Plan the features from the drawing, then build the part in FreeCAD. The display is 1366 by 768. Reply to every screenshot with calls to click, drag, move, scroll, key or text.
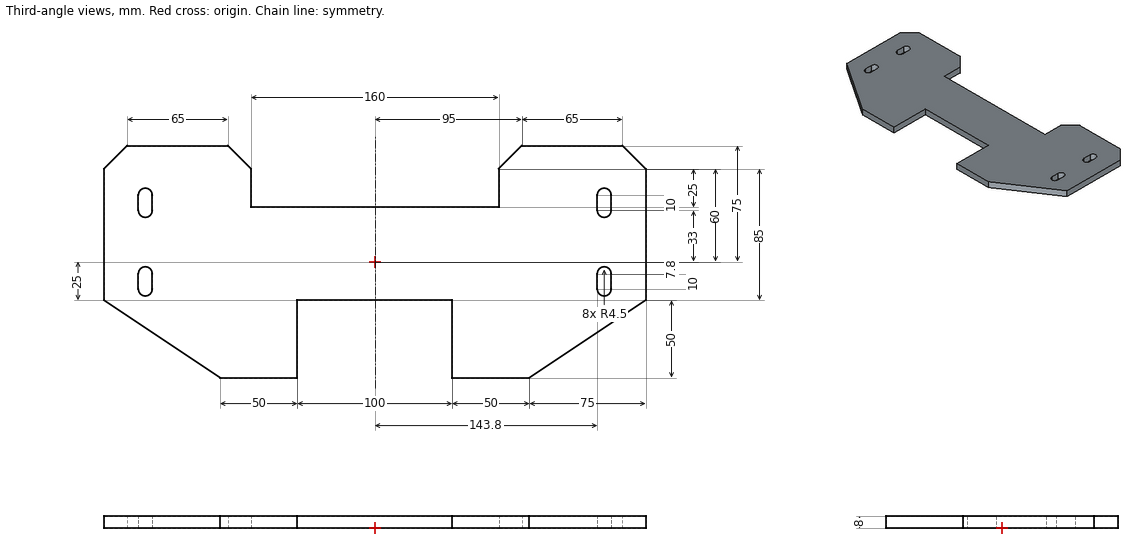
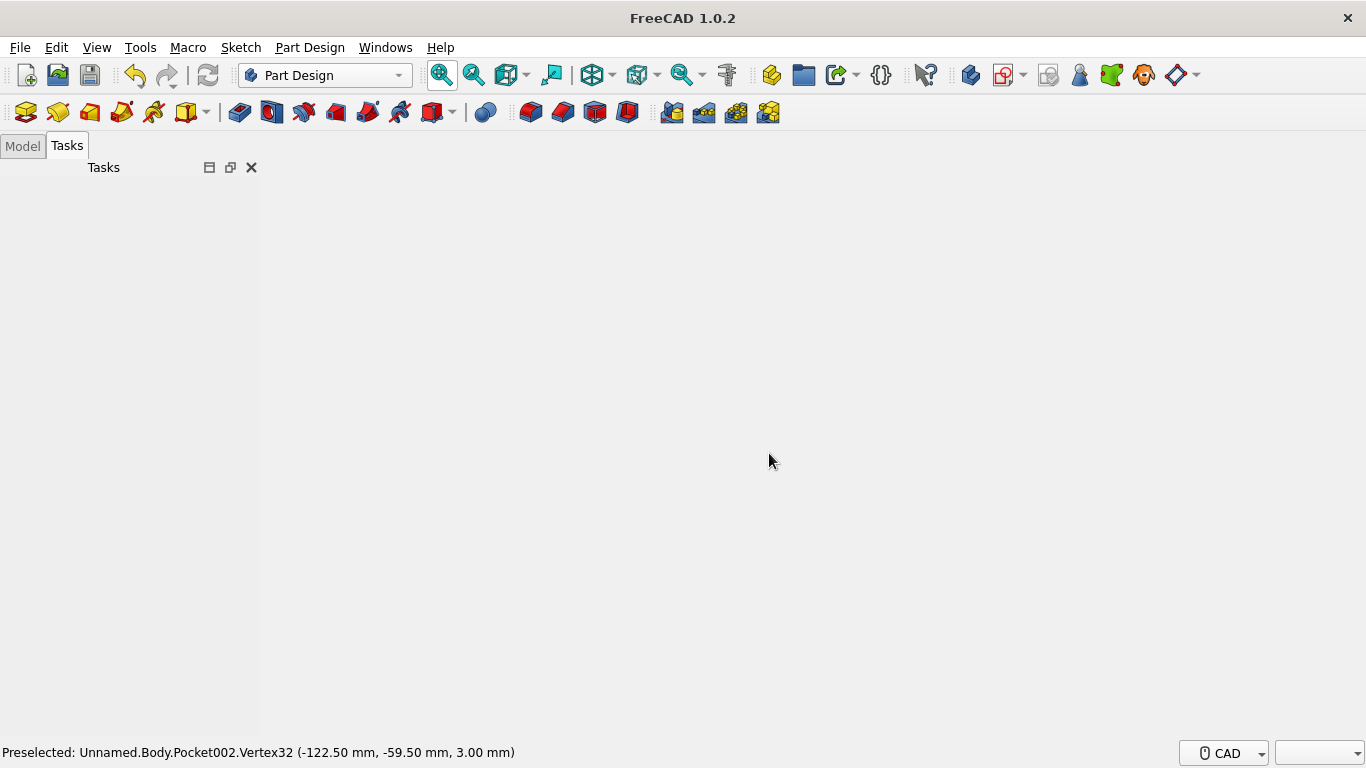
click(26, 76)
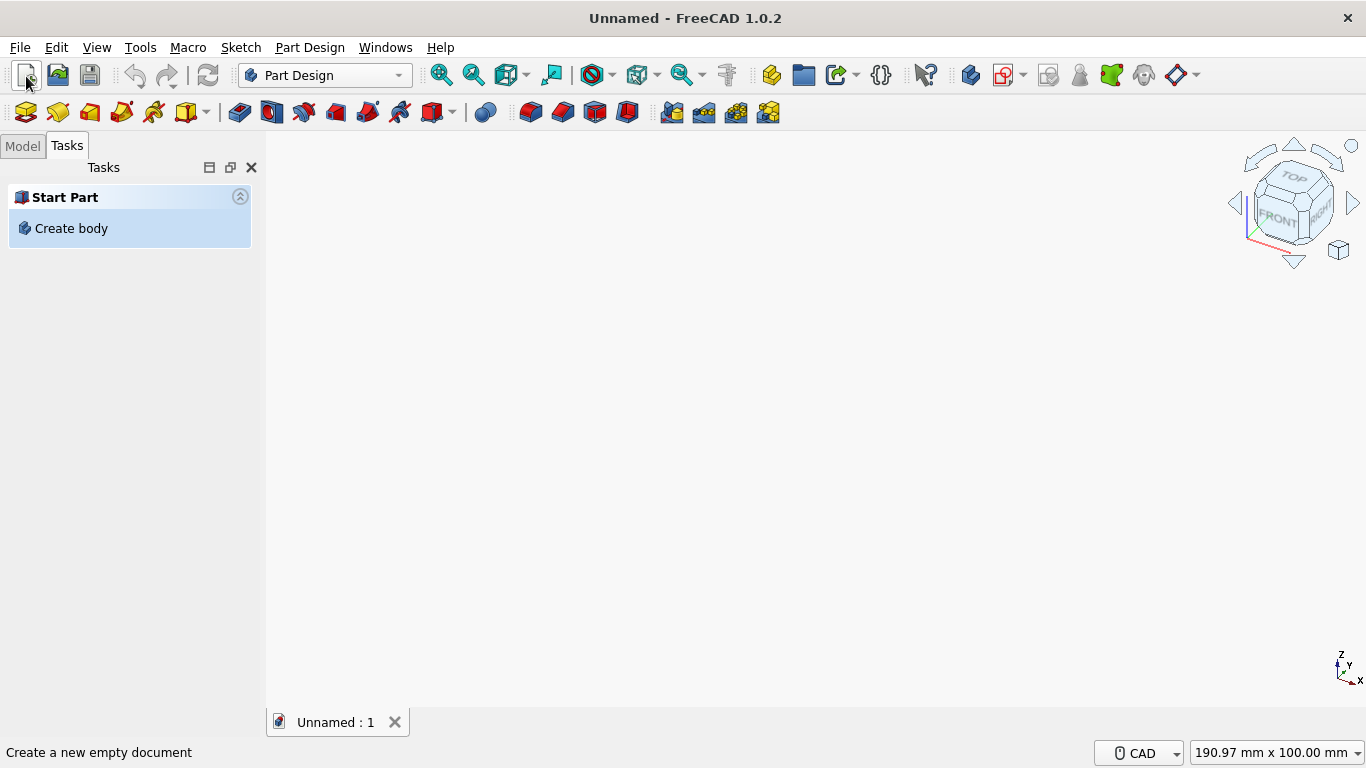
click(1004, 76)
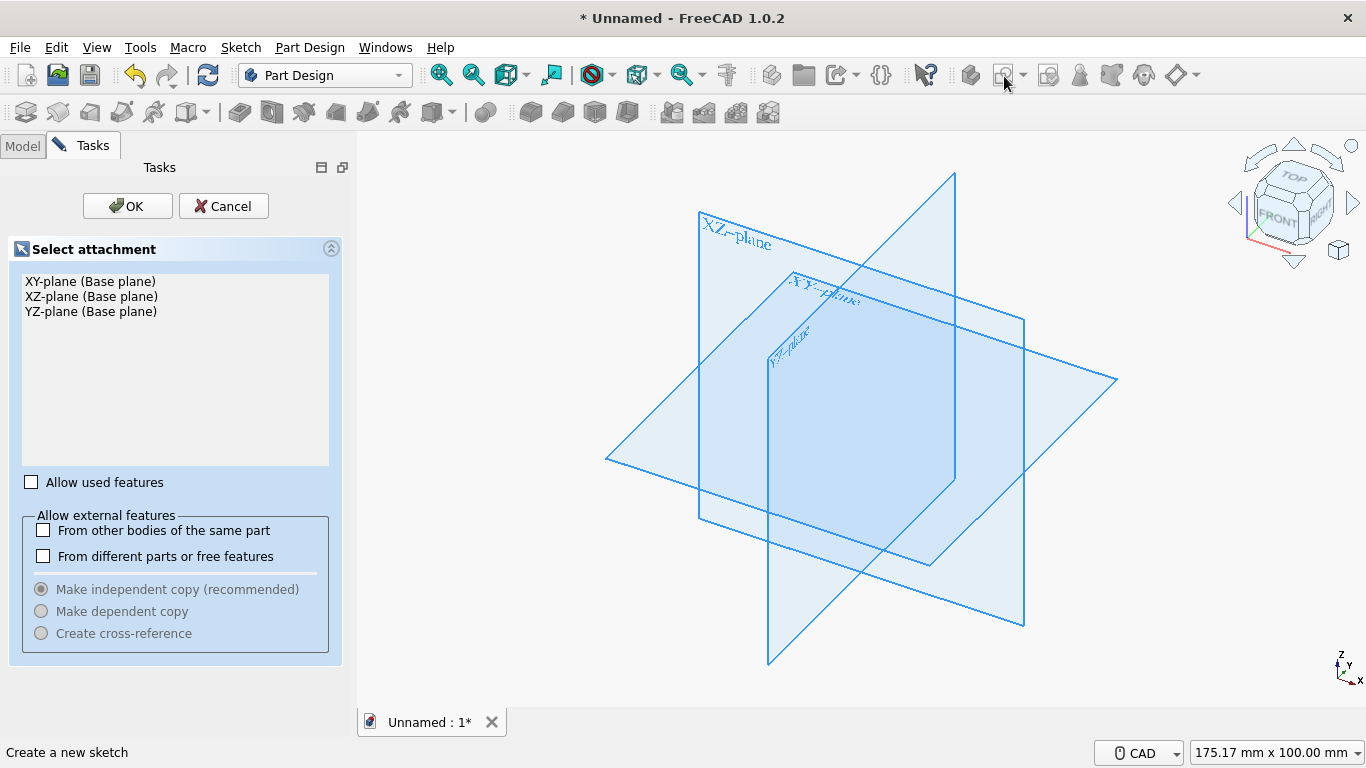
click(82, 282)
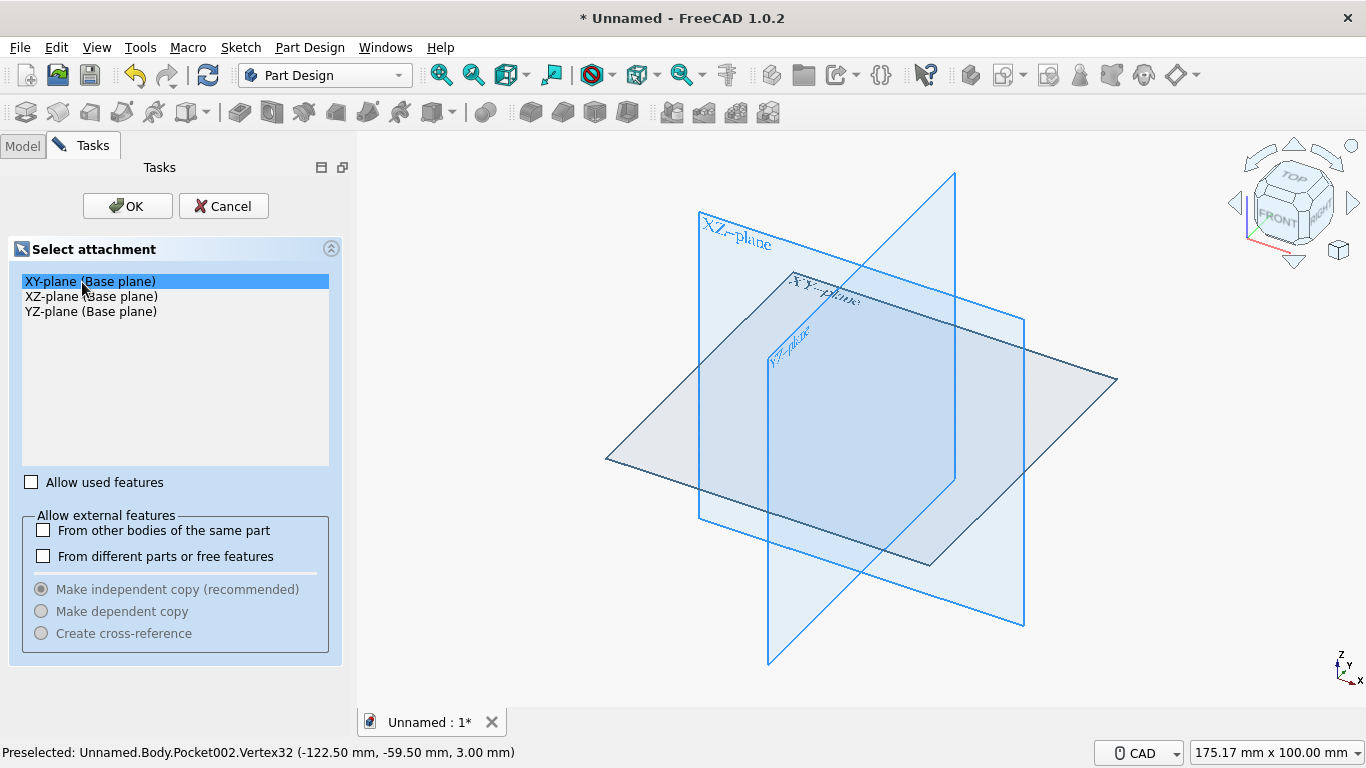
click(128, 206)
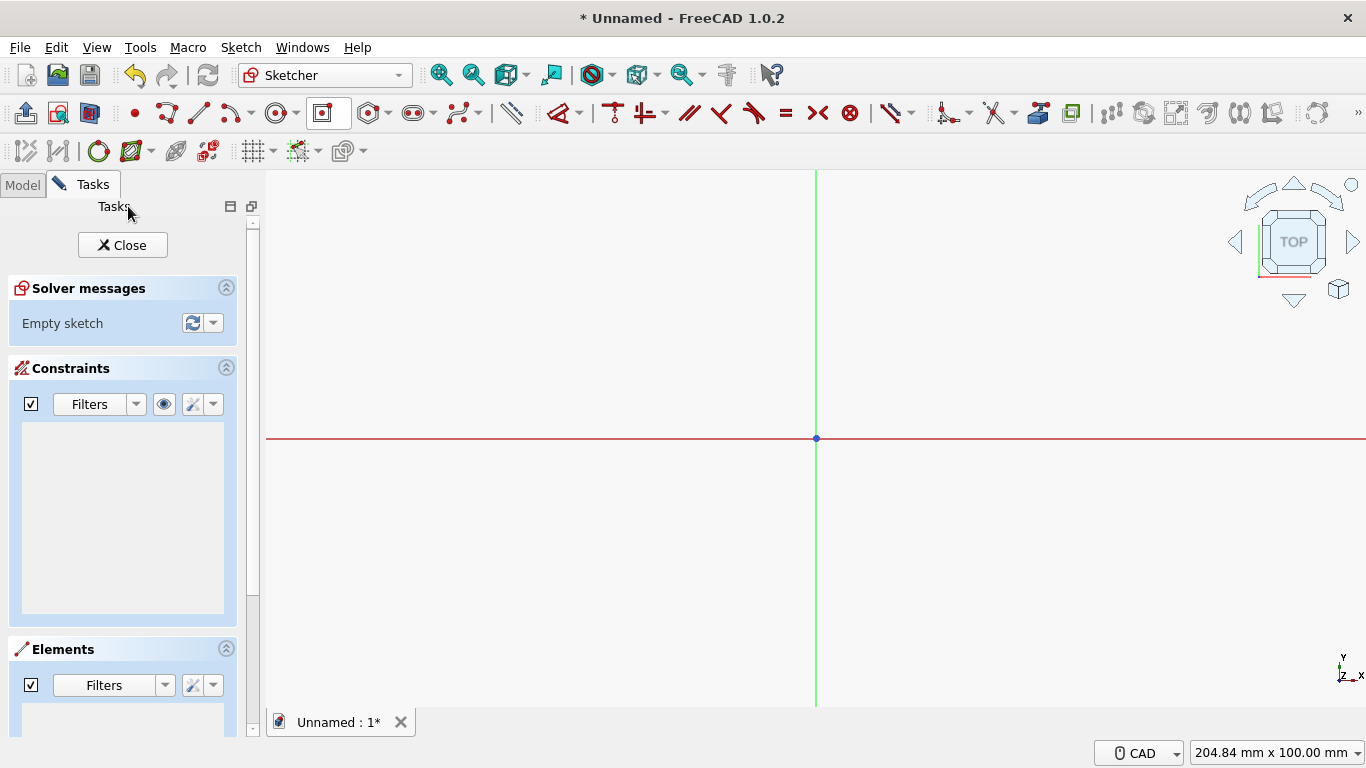
scroll(708, 439, down, 5)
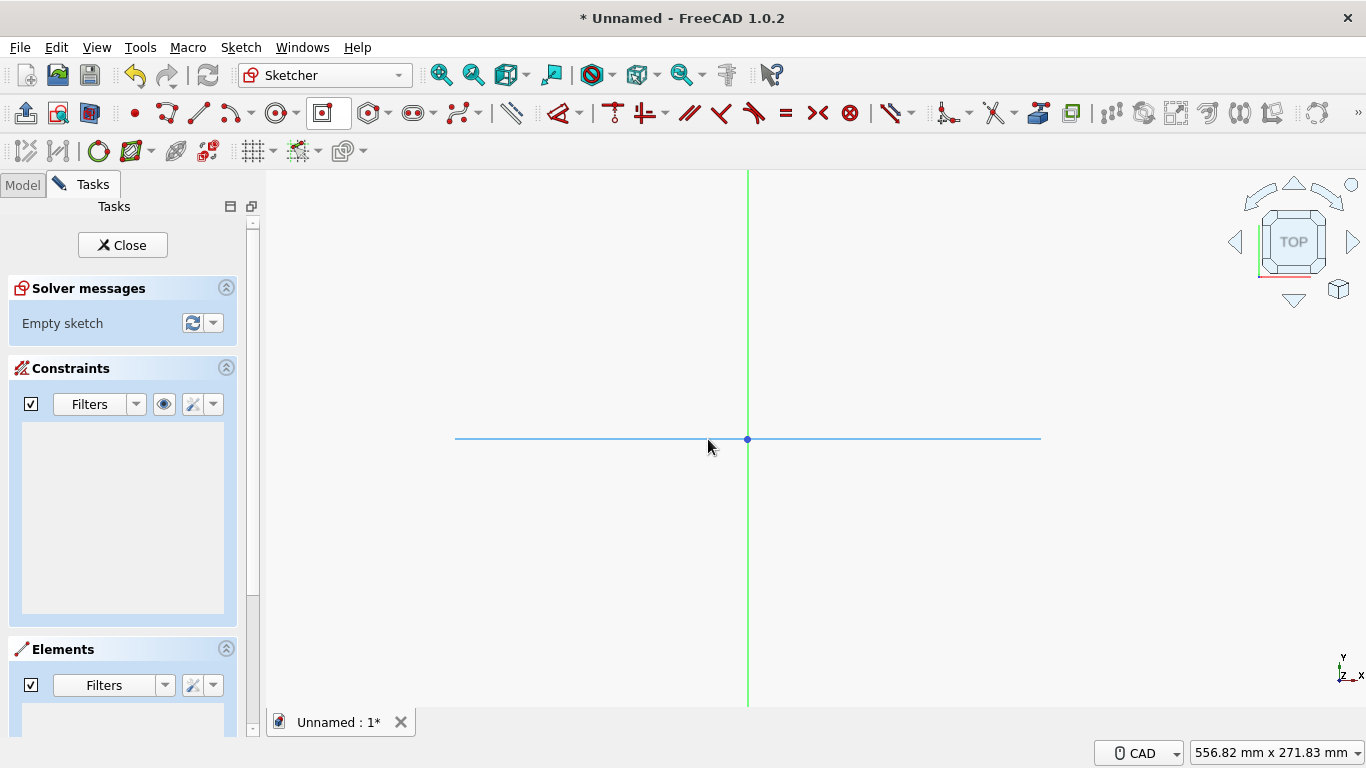
click(168, 114)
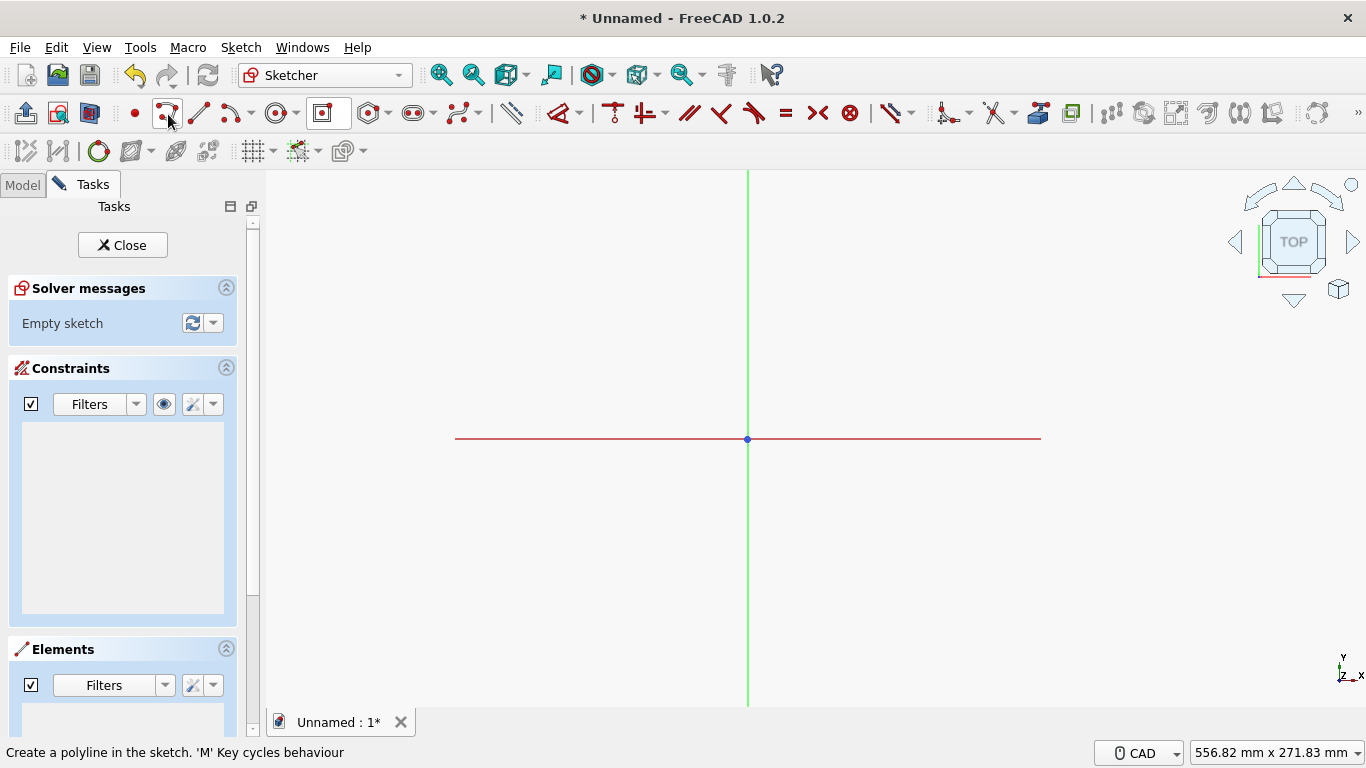
click(649, 489)
click(847, 489)
click(847, 587)
click(946, 587)
click(1094, 489)
click(1094, 321)
click(1064, 291)
click(936, 291)
click(906, 321)
click(906, 370)
click(590, 370)
click(590, 321)
click(560, 291)
click(432, 291)
click(402, 321)
click(402, 489)
click(550, 587)
click(649, 587)
click(649, 490)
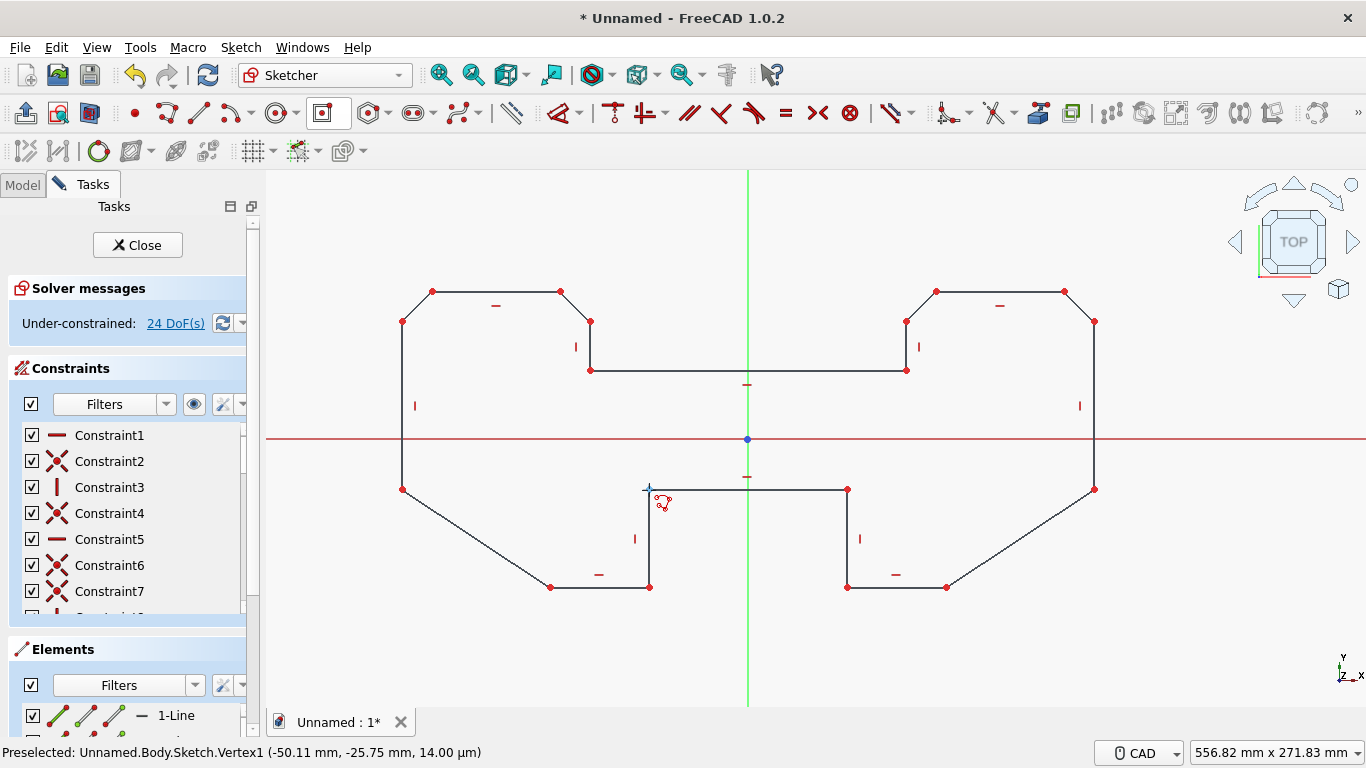
click(414, 114)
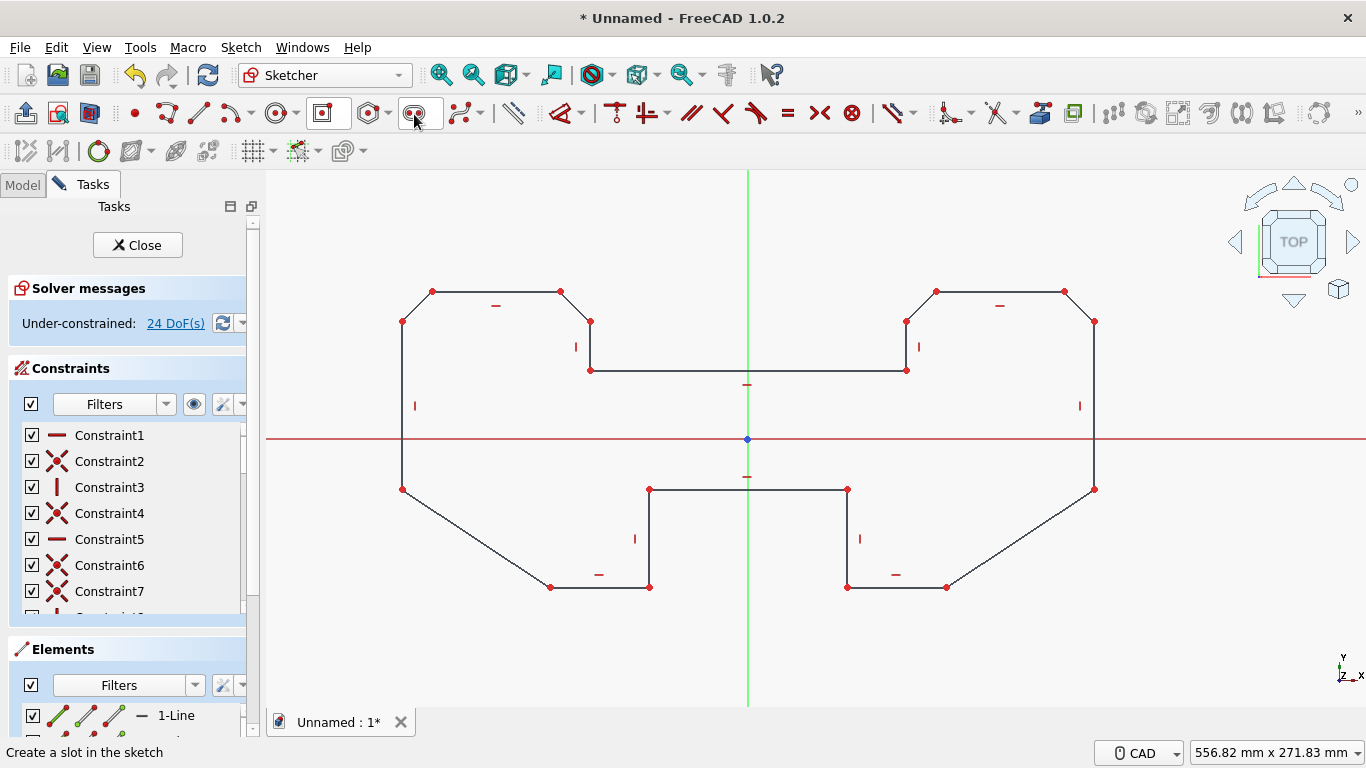
scroll(1041, 474, up, 5)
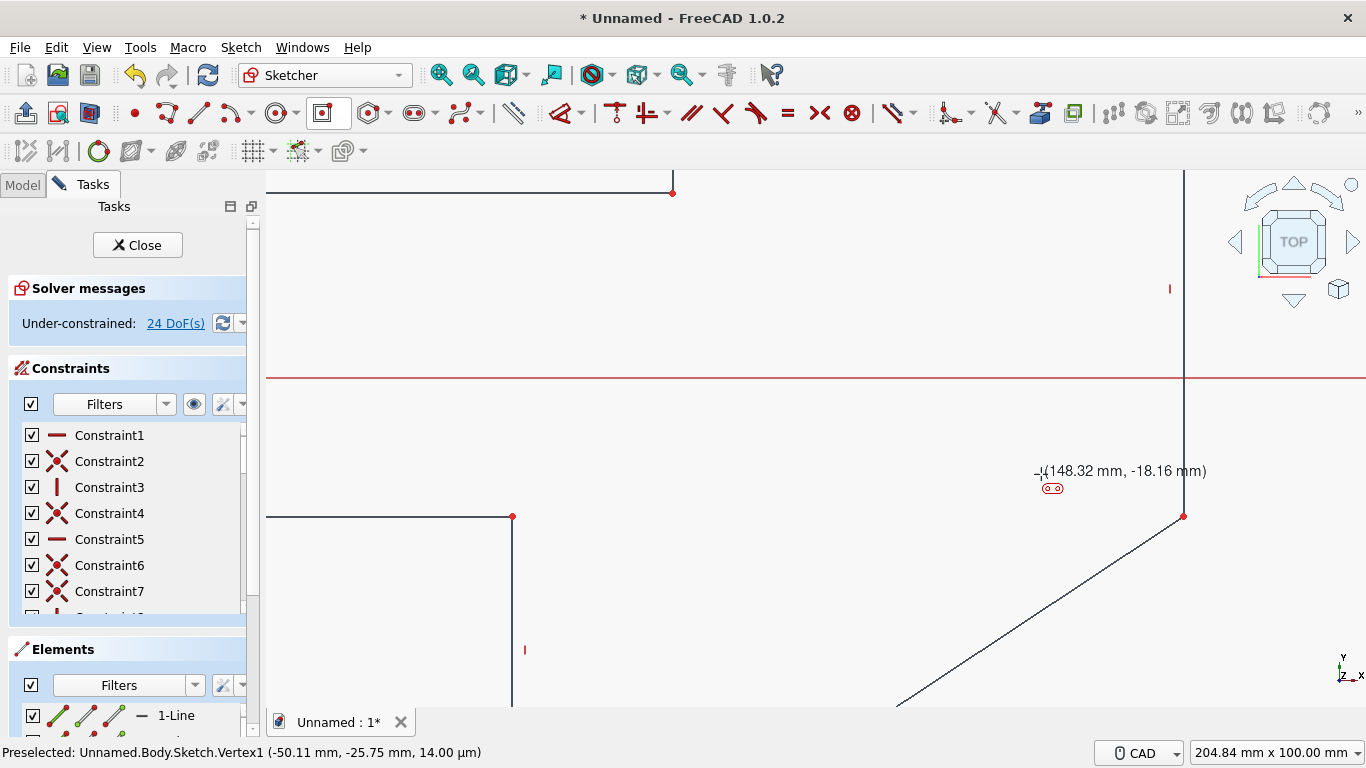
click(1040, 474)